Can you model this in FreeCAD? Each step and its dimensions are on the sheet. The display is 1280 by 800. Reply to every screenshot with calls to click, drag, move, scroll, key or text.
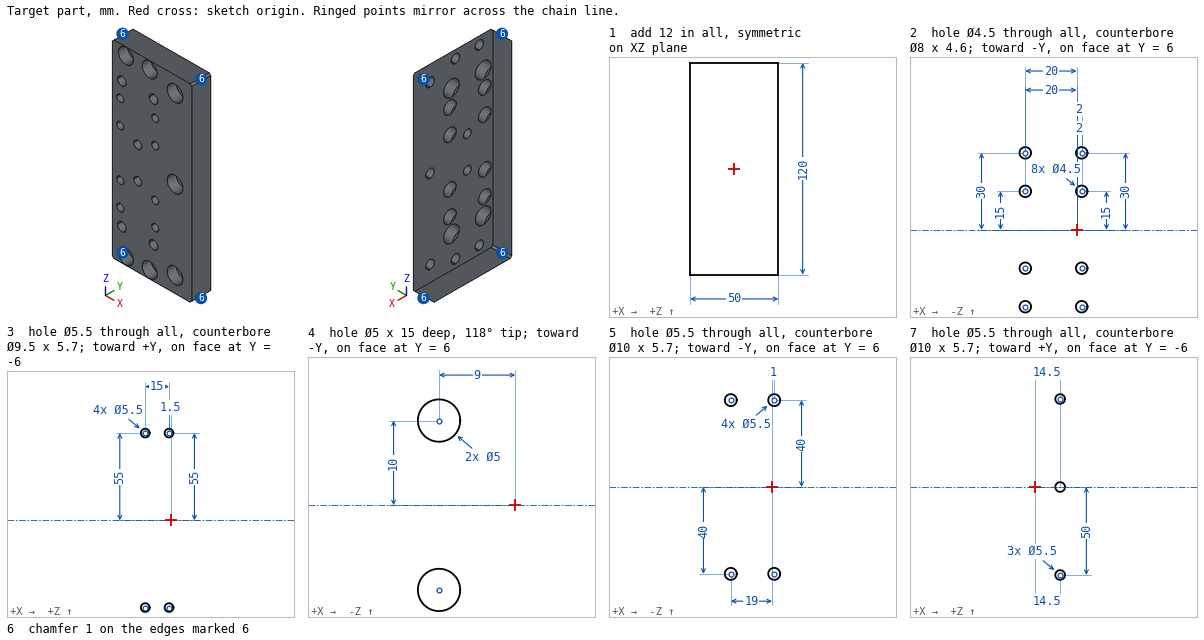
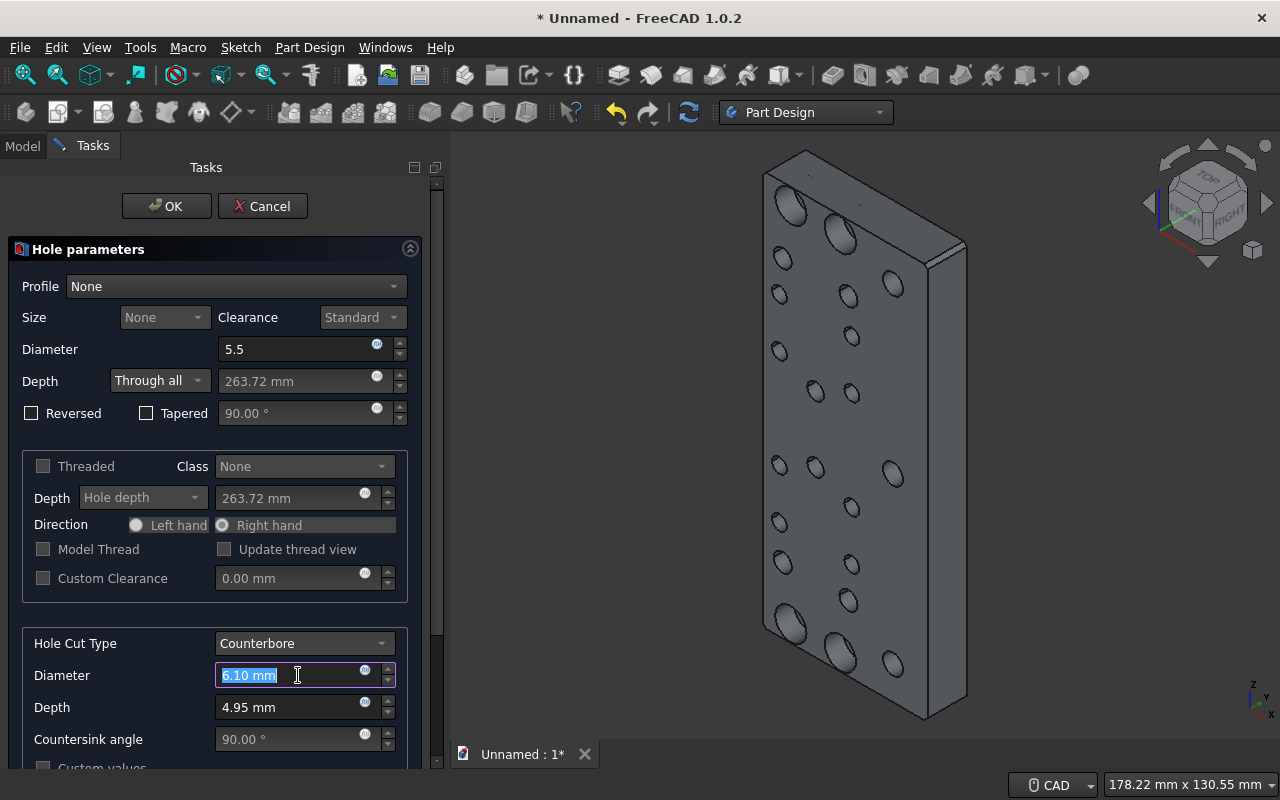
text(10)
key(Tab)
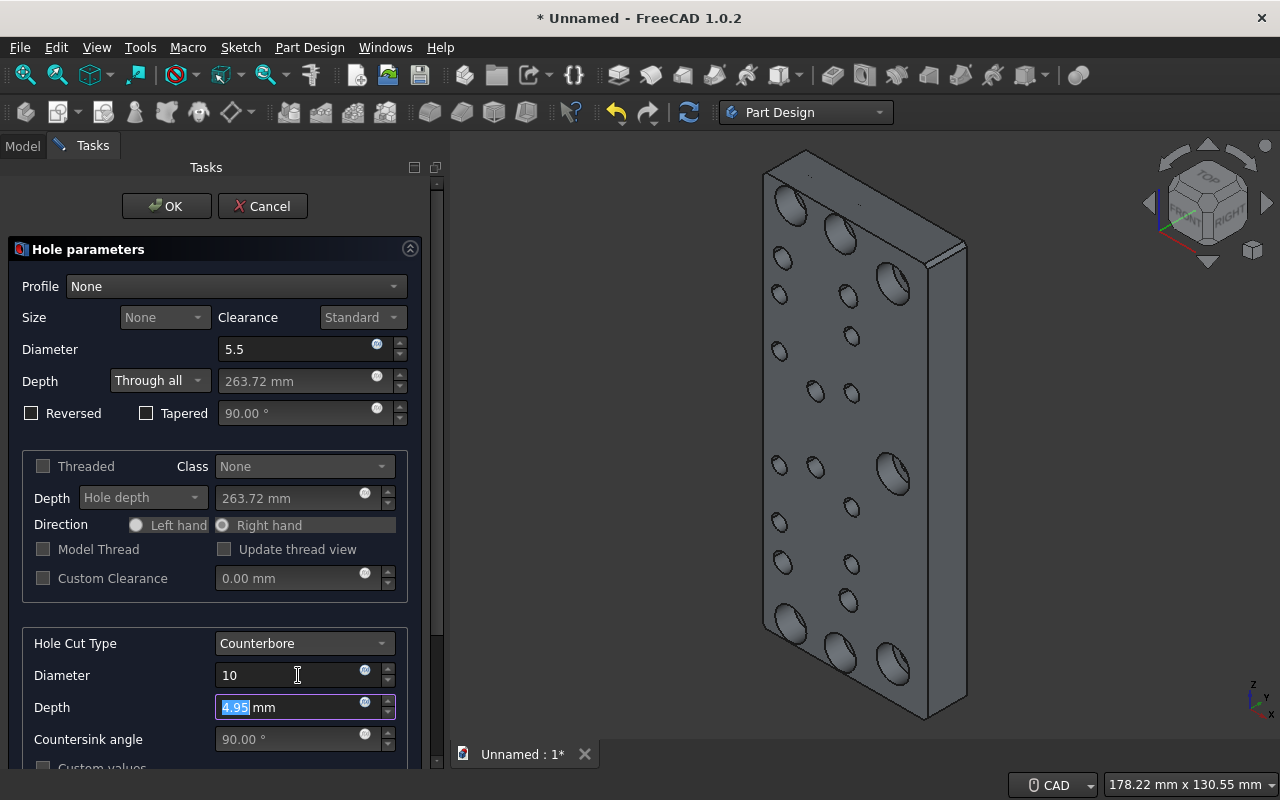
text(5.7)
key(Tab)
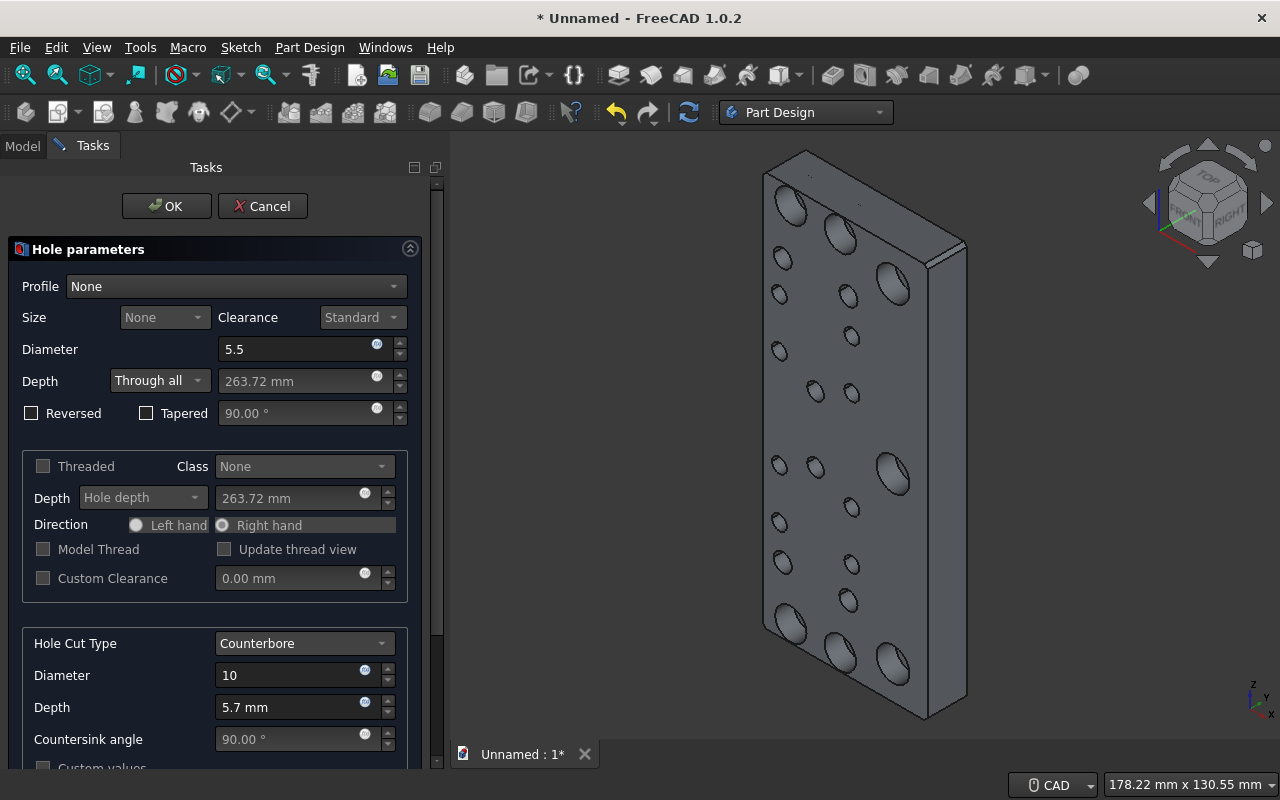
click(167, 206)